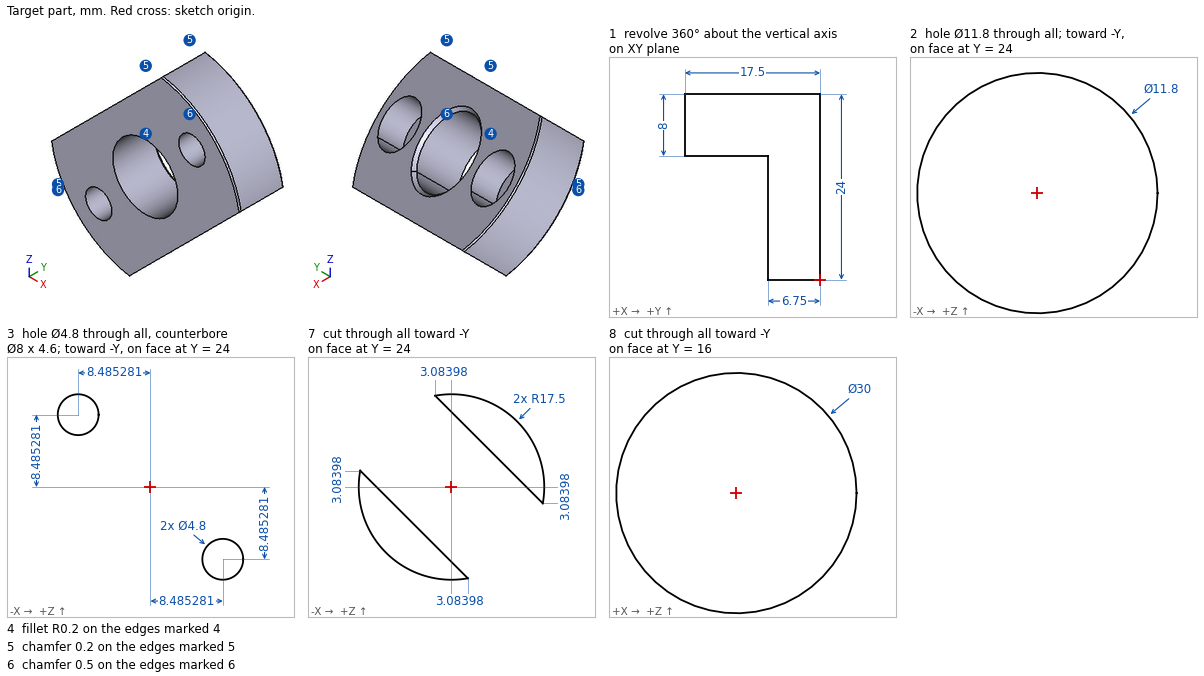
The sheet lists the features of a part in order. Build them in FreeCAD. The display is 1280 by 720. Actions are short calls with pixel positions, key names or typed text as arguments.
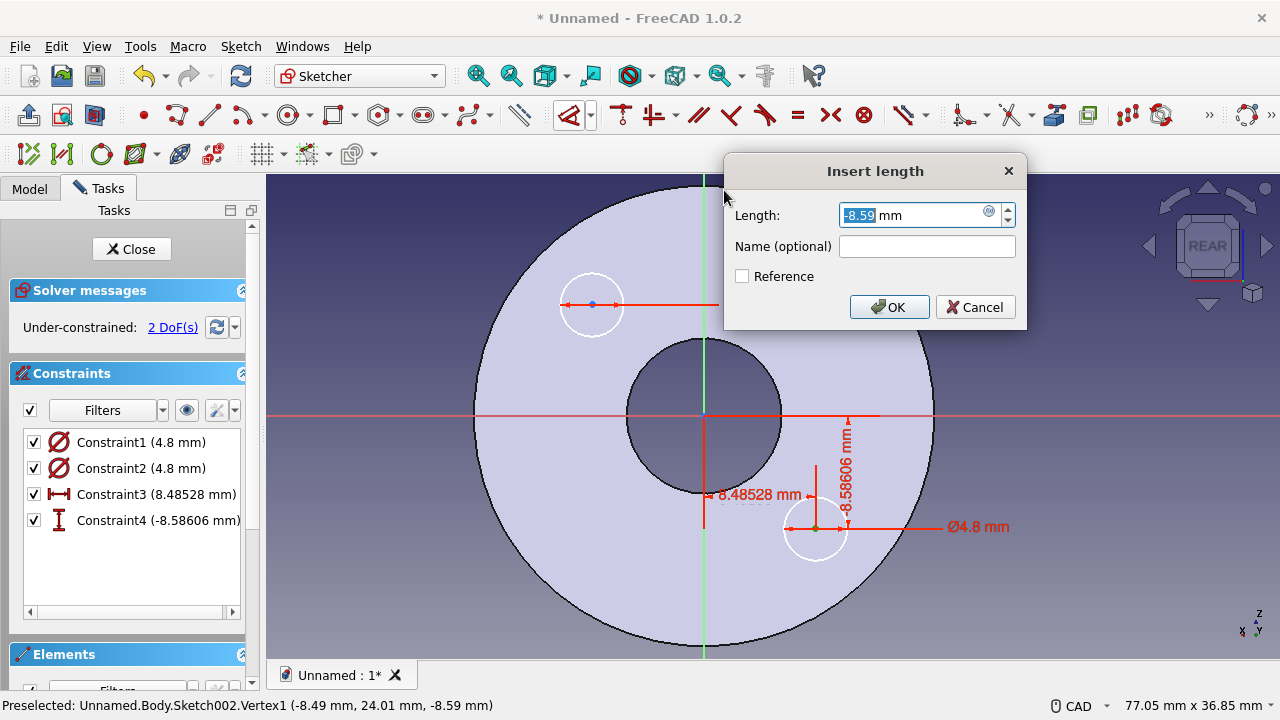
text(-8.485281)
key(Return)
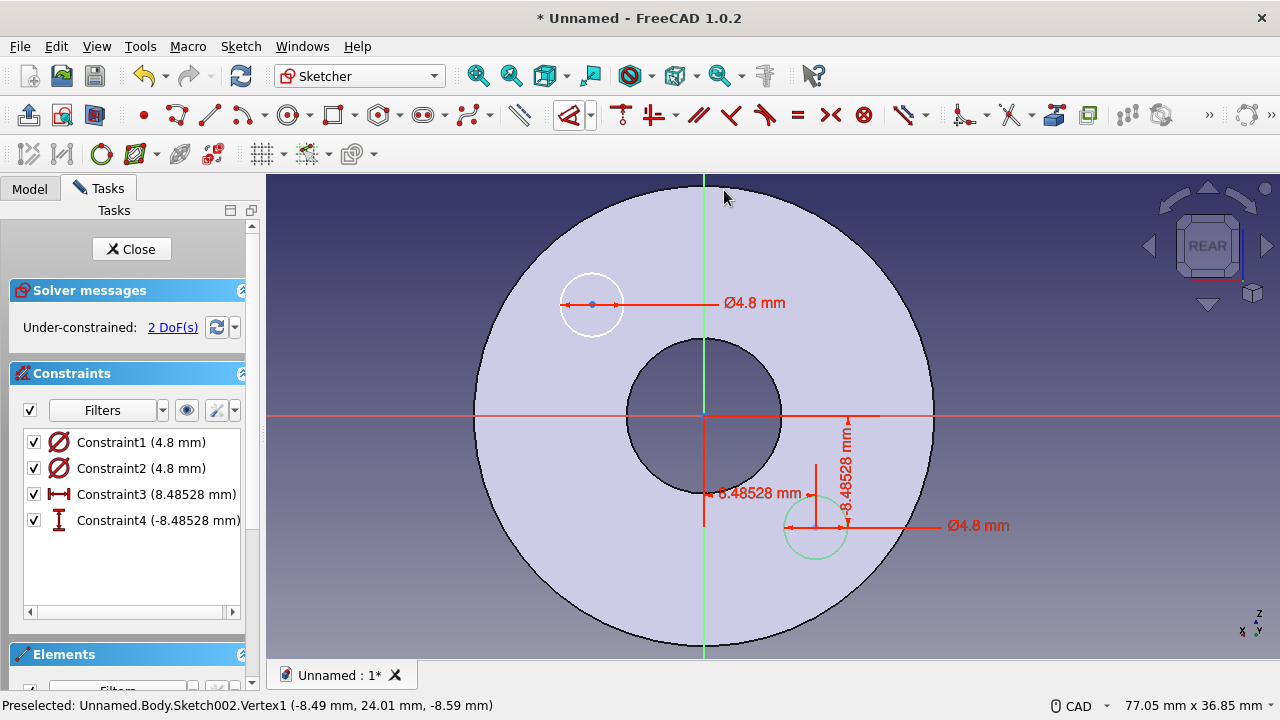
click(592, 305)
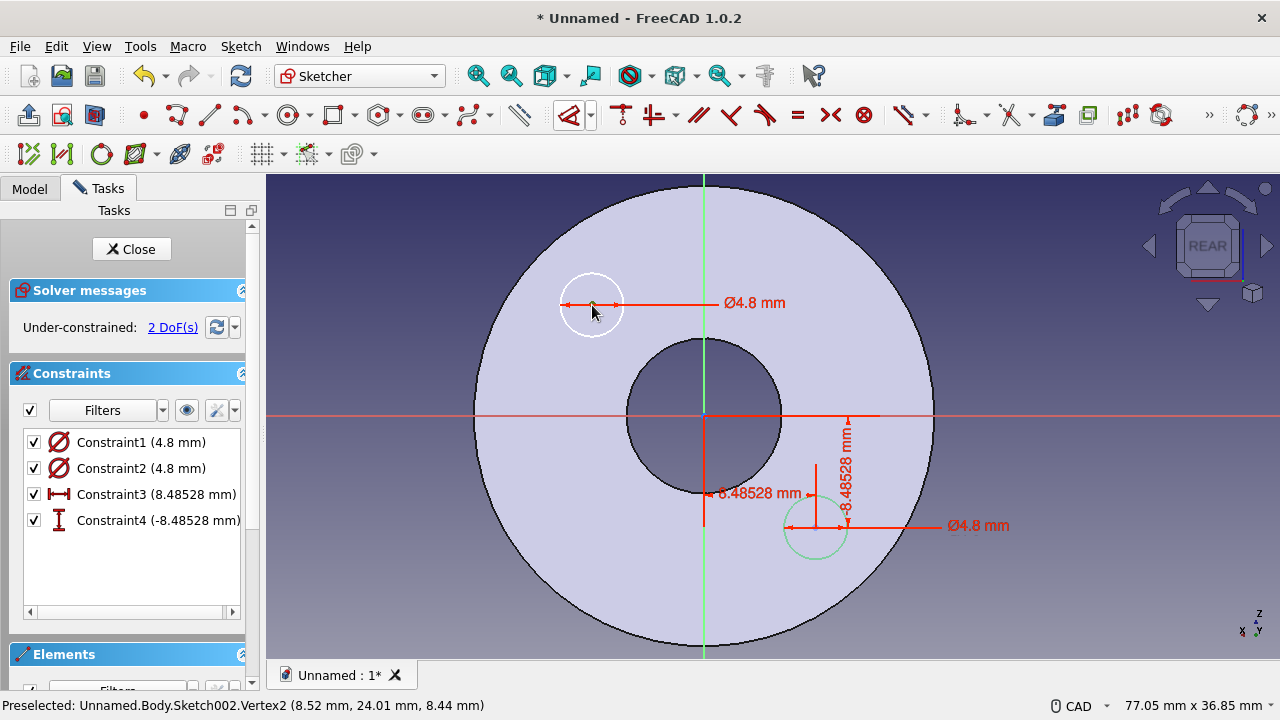
click(590, 116)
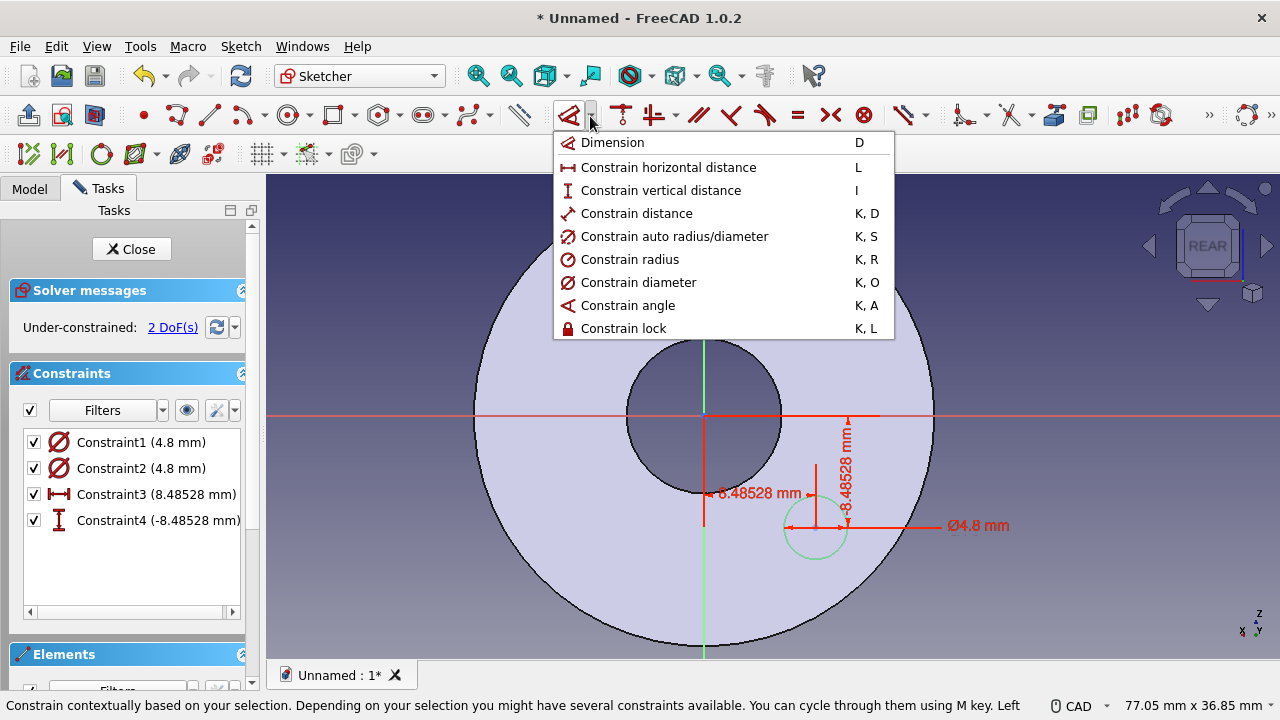
click(724, 168)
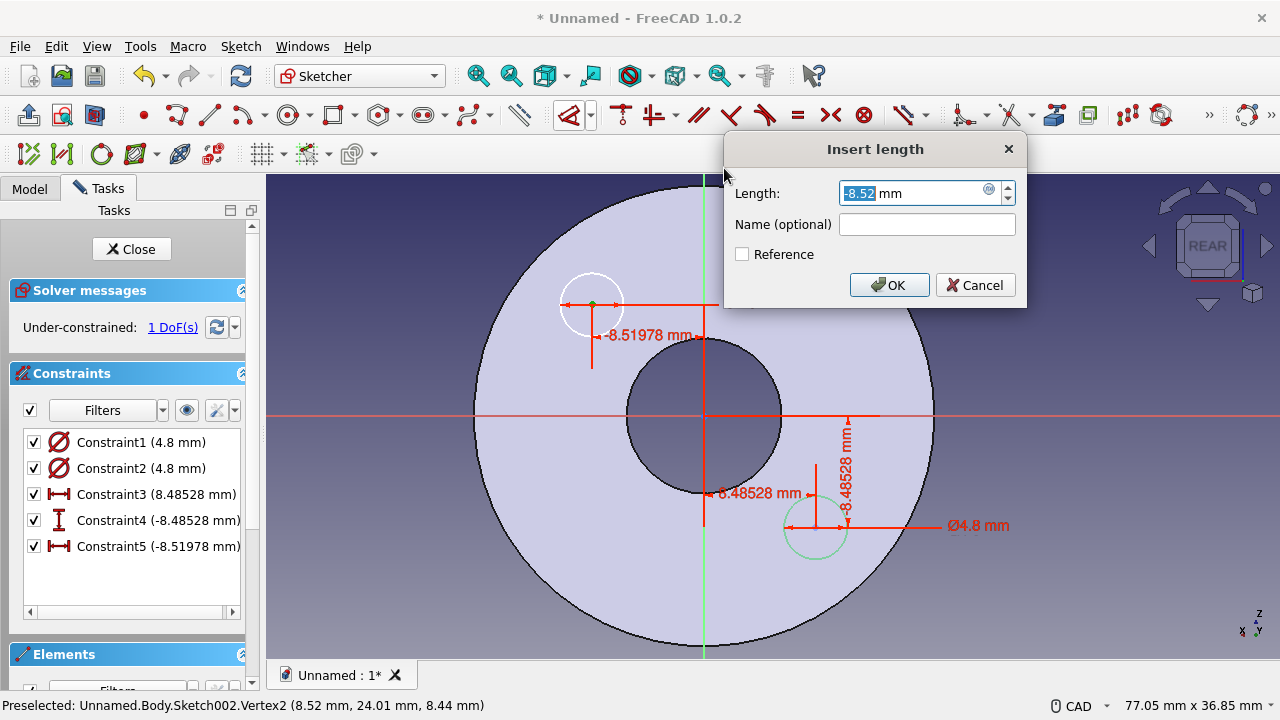
text(-8.485281)
key(Return)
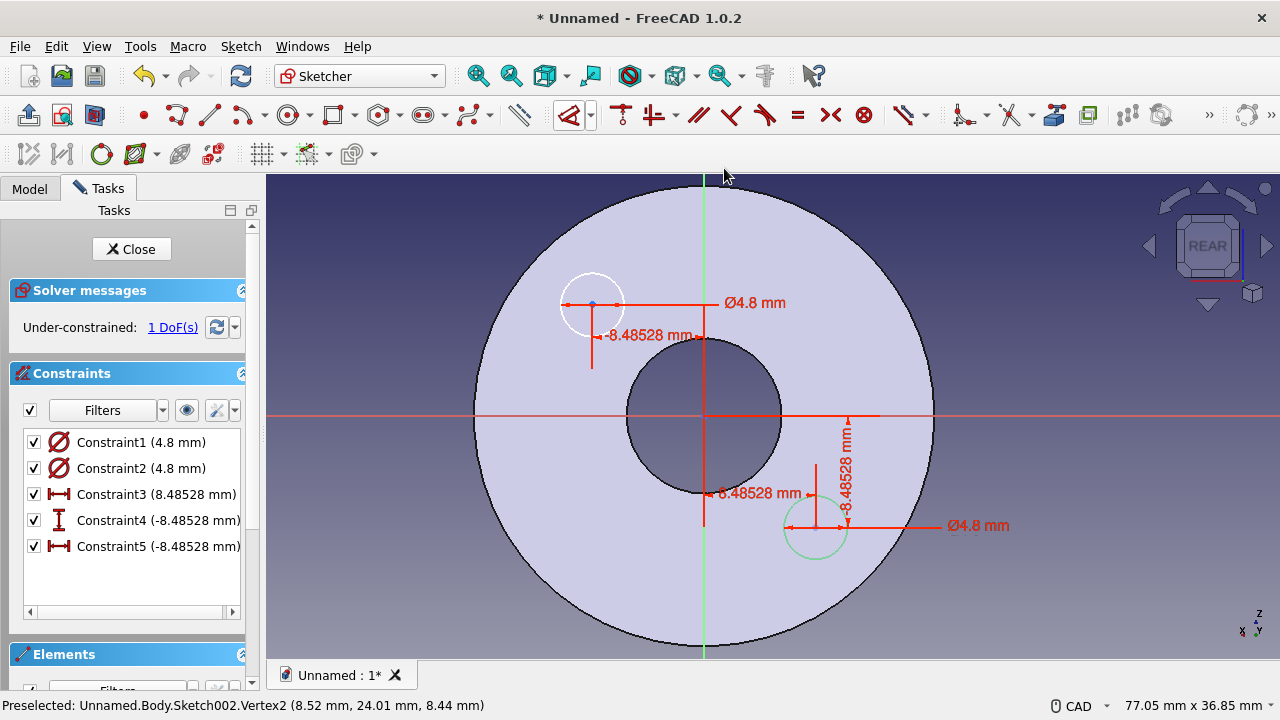
click(592, 305)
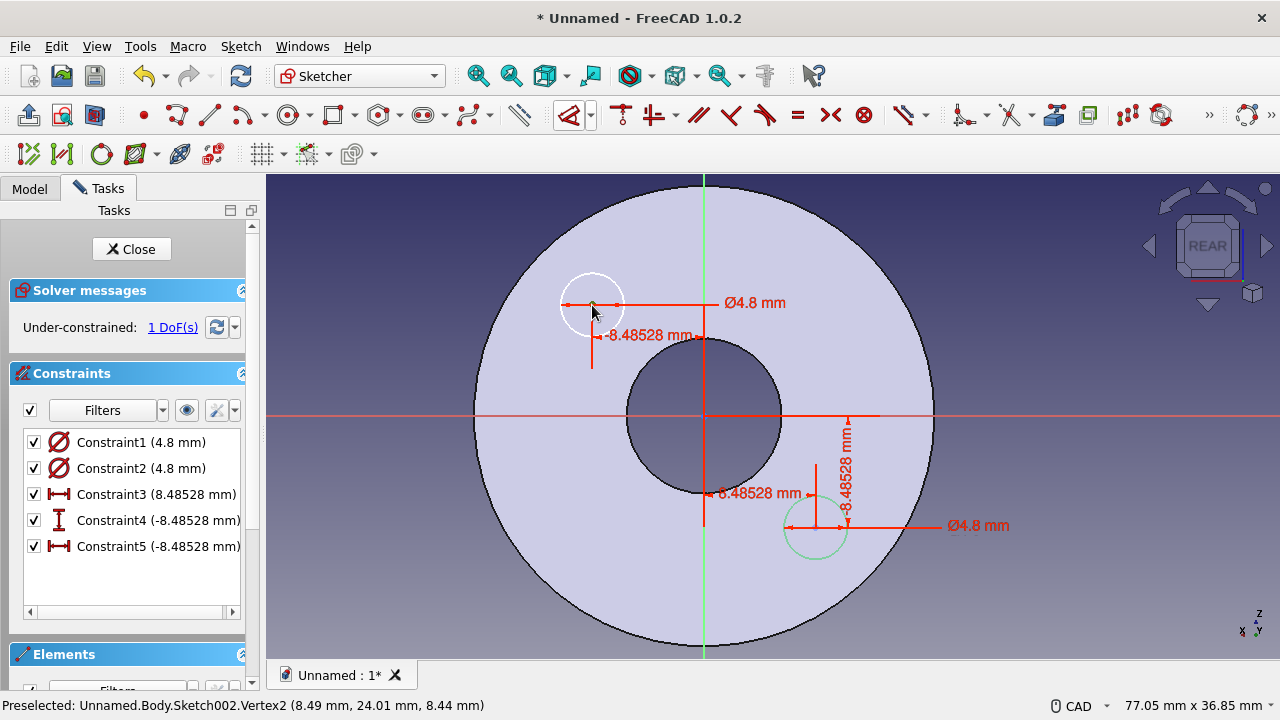
key(i)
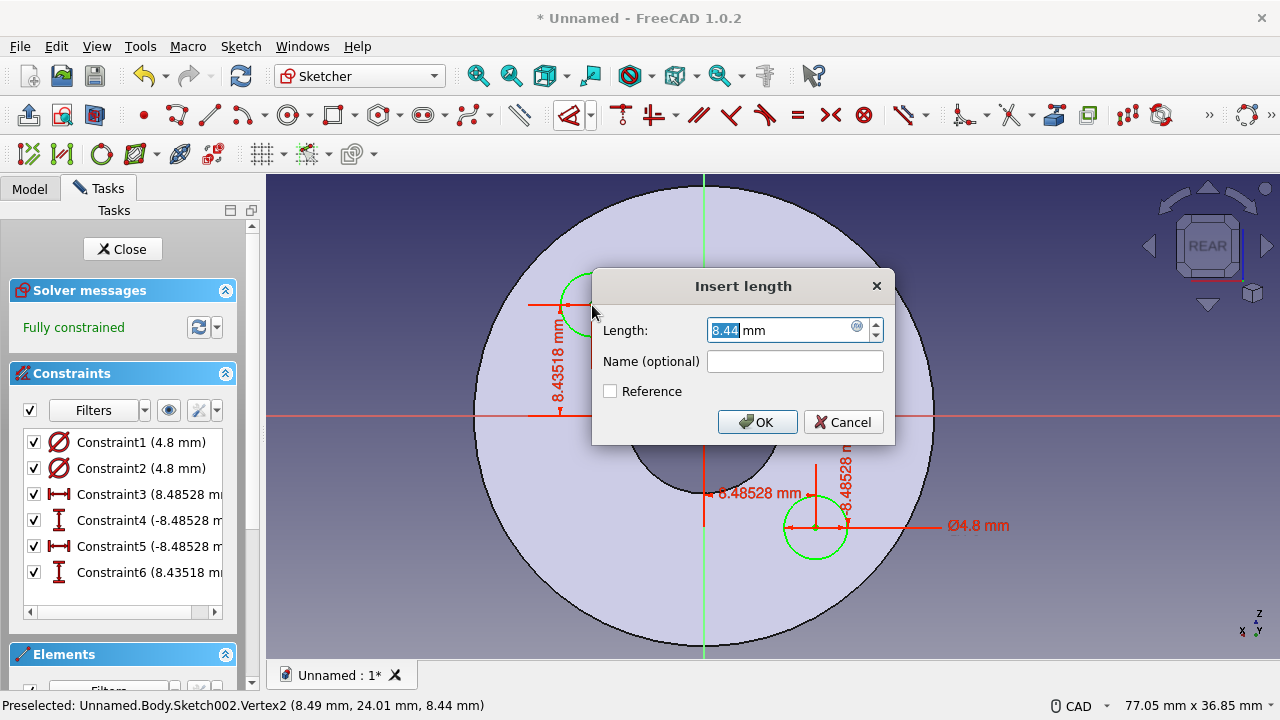
text(8.485281)
key(Return)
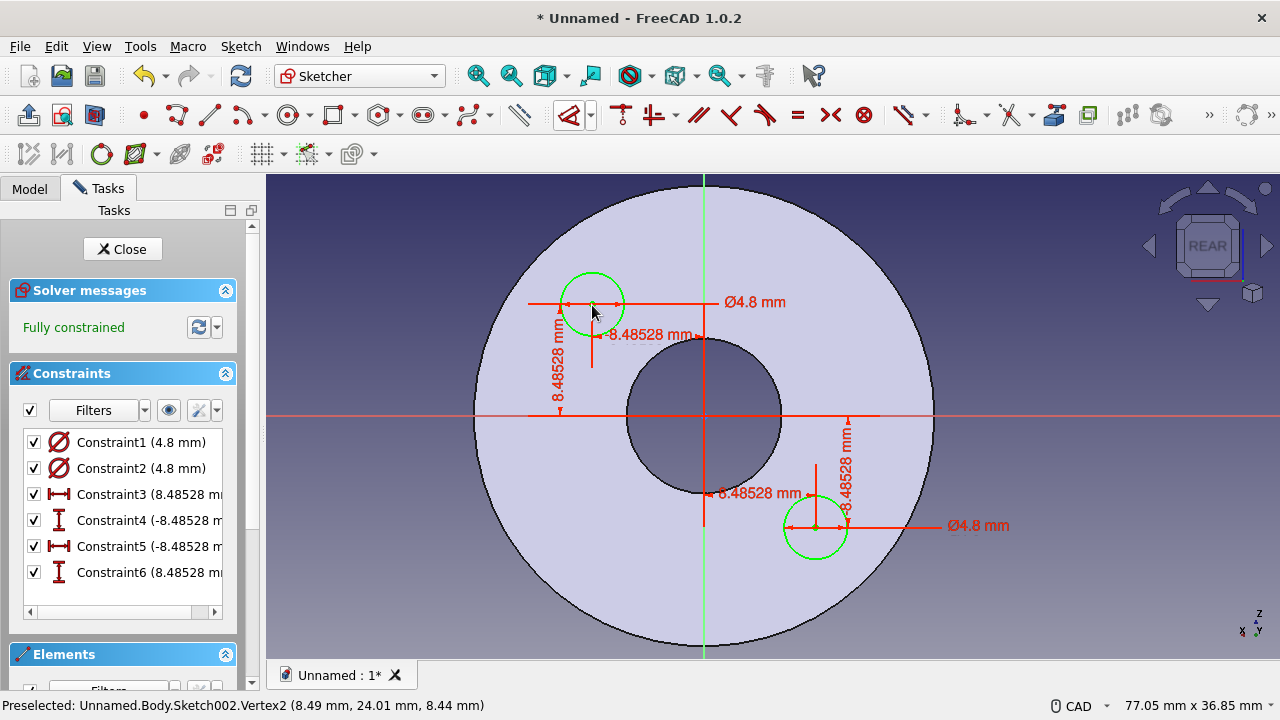
click(123, 249)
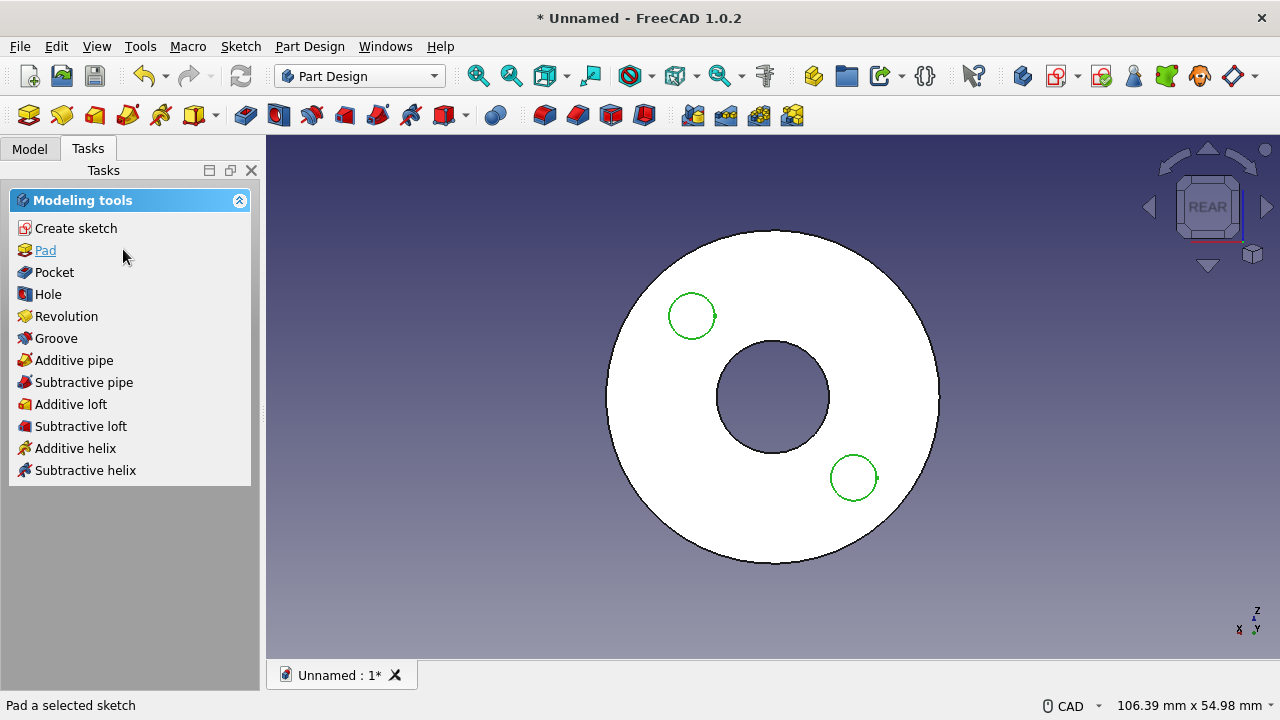
click(279, 116)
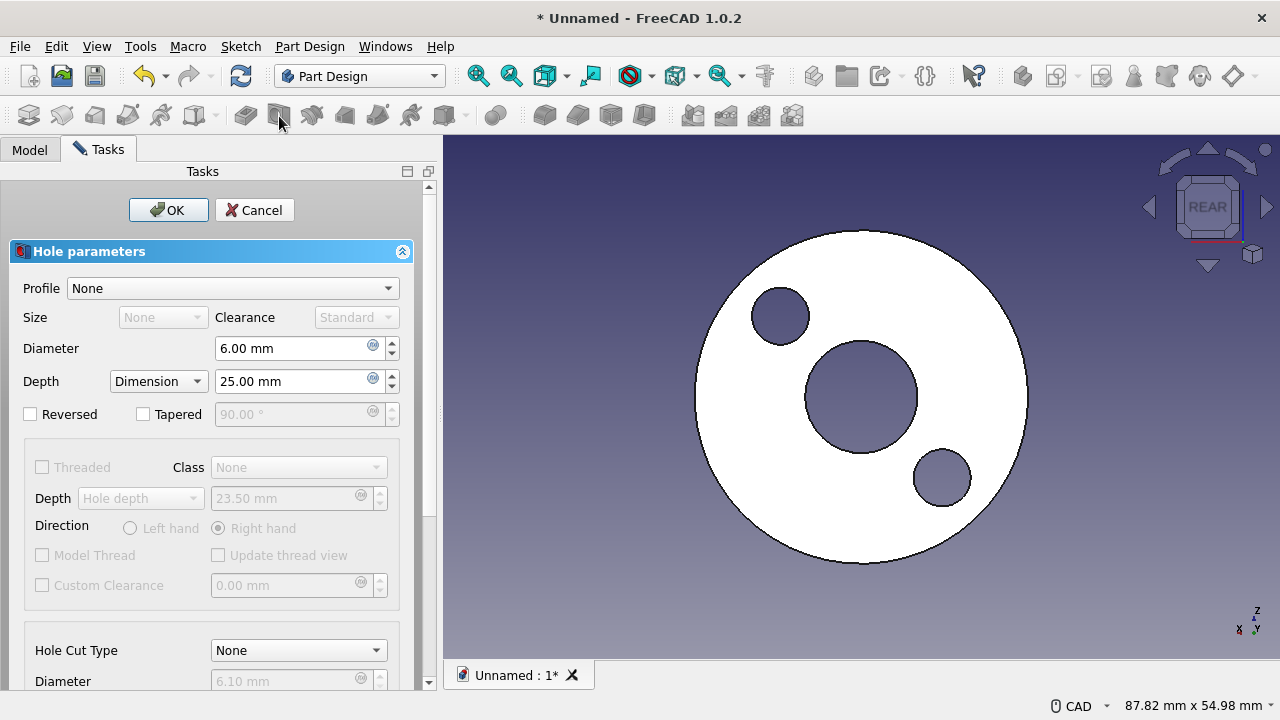
triple_click(300, 348)